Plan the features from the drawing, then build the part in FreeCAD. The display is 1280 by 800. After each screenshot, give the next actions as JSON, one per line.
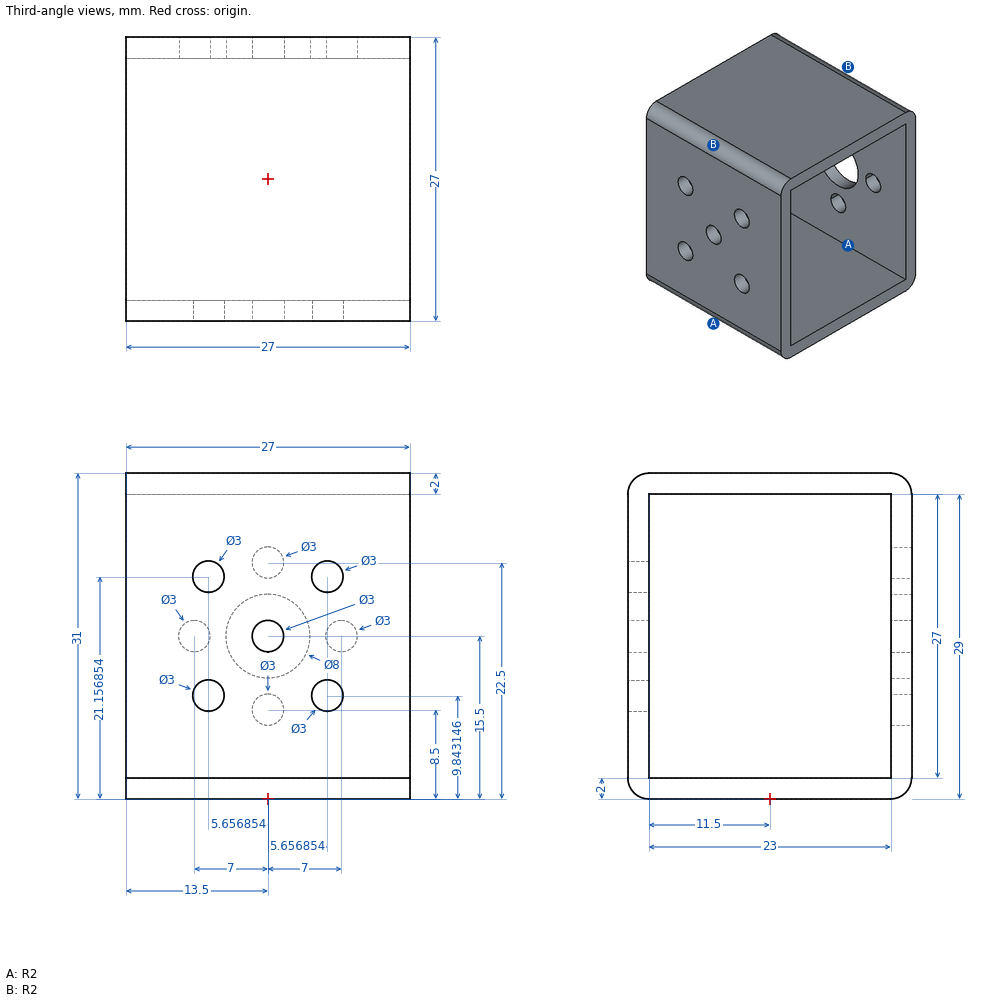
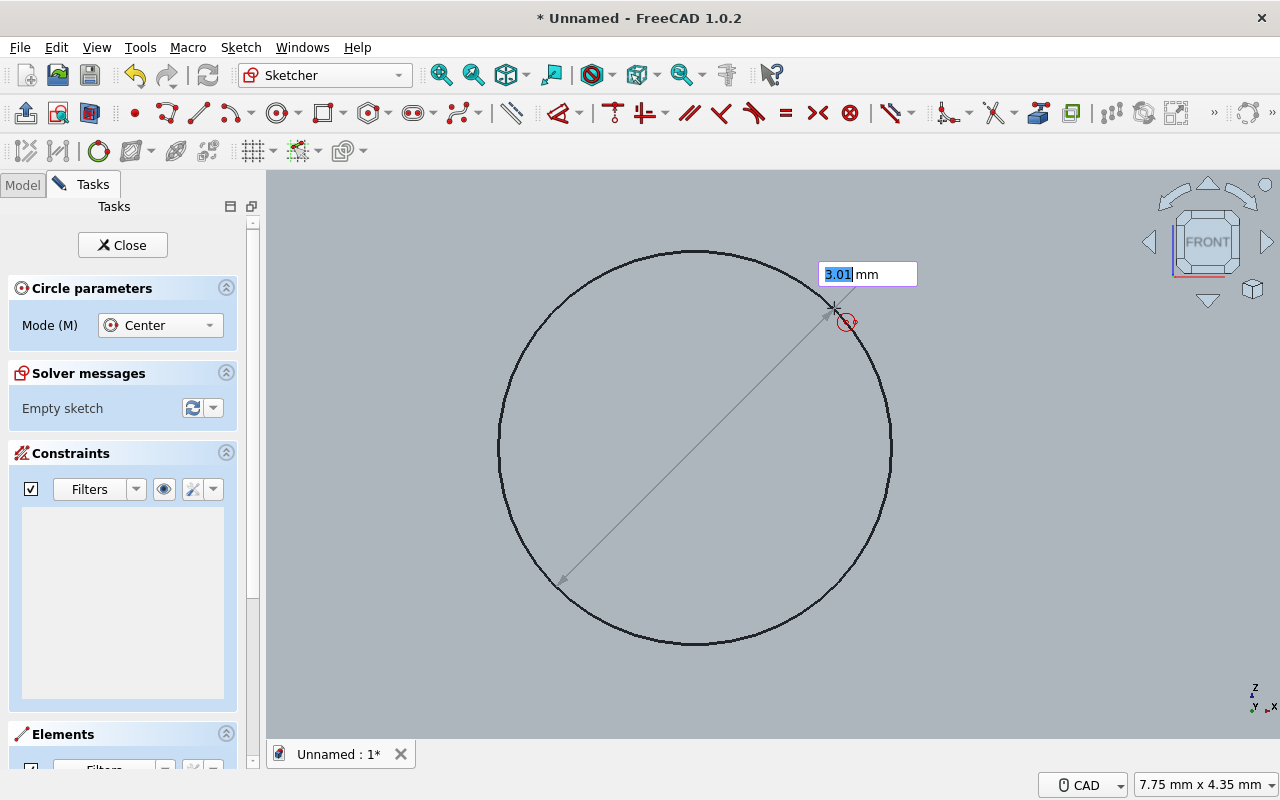
{"action": "type", "text": "3"}
{"action": "key", "text": "Return"}
{"action": "key", "text": "Escape"}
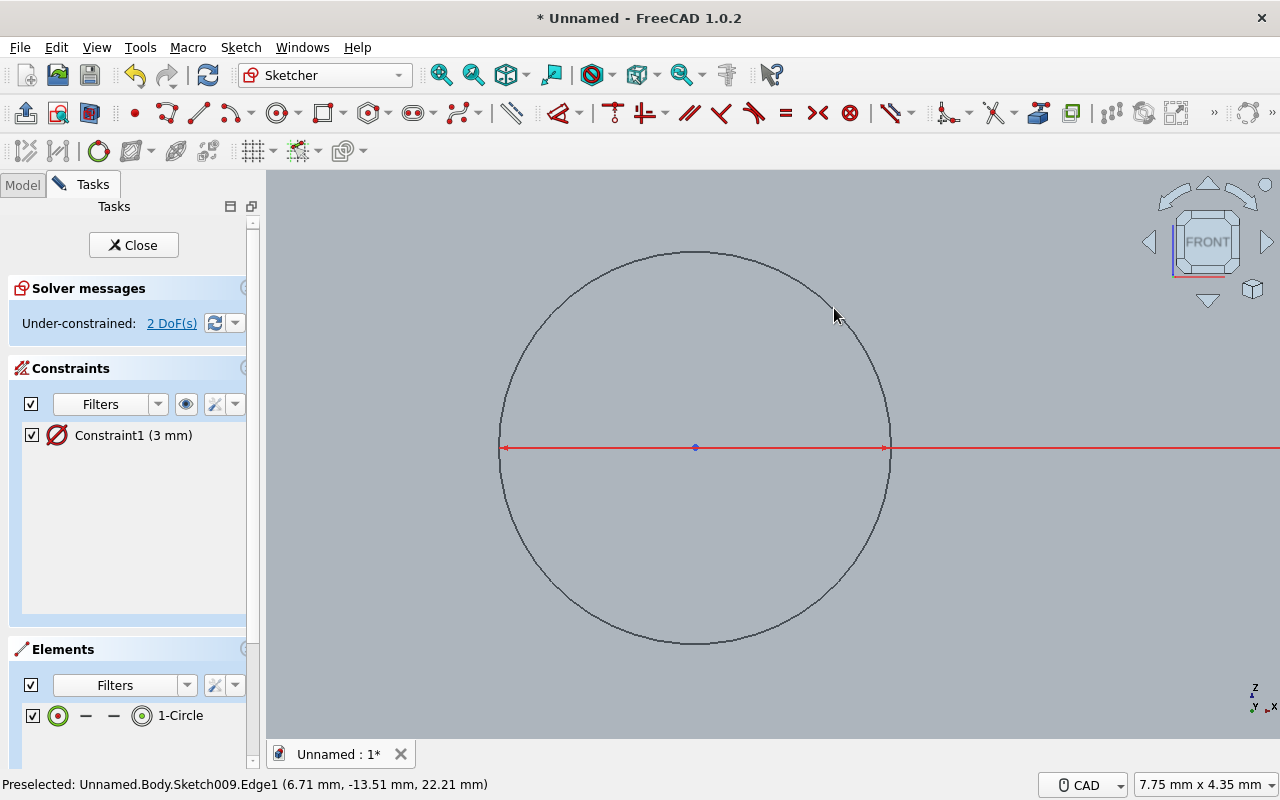
{"action": "left_click", "coordinate": [558, 114]}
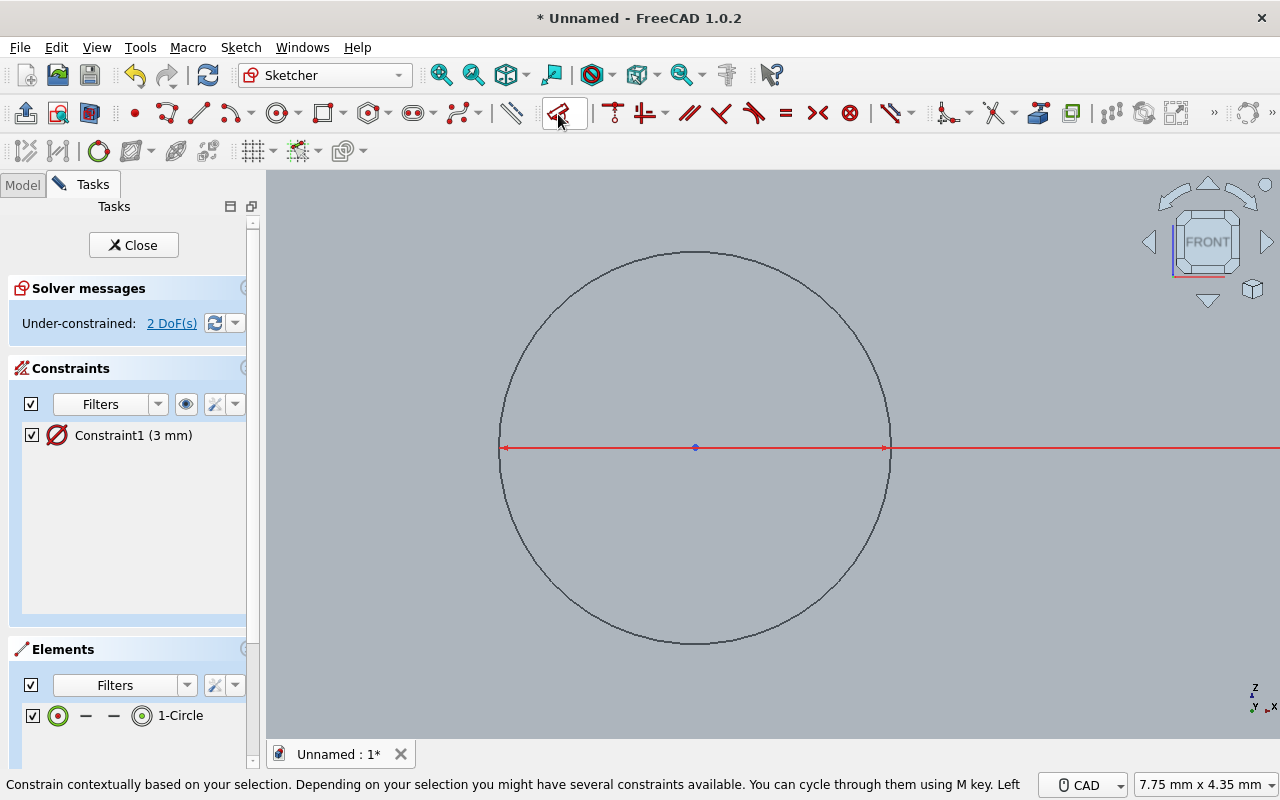
{"action": "left_click", "coordinate": [695, 448]}
{"action": "left_click", "coordinate": [402, 414]}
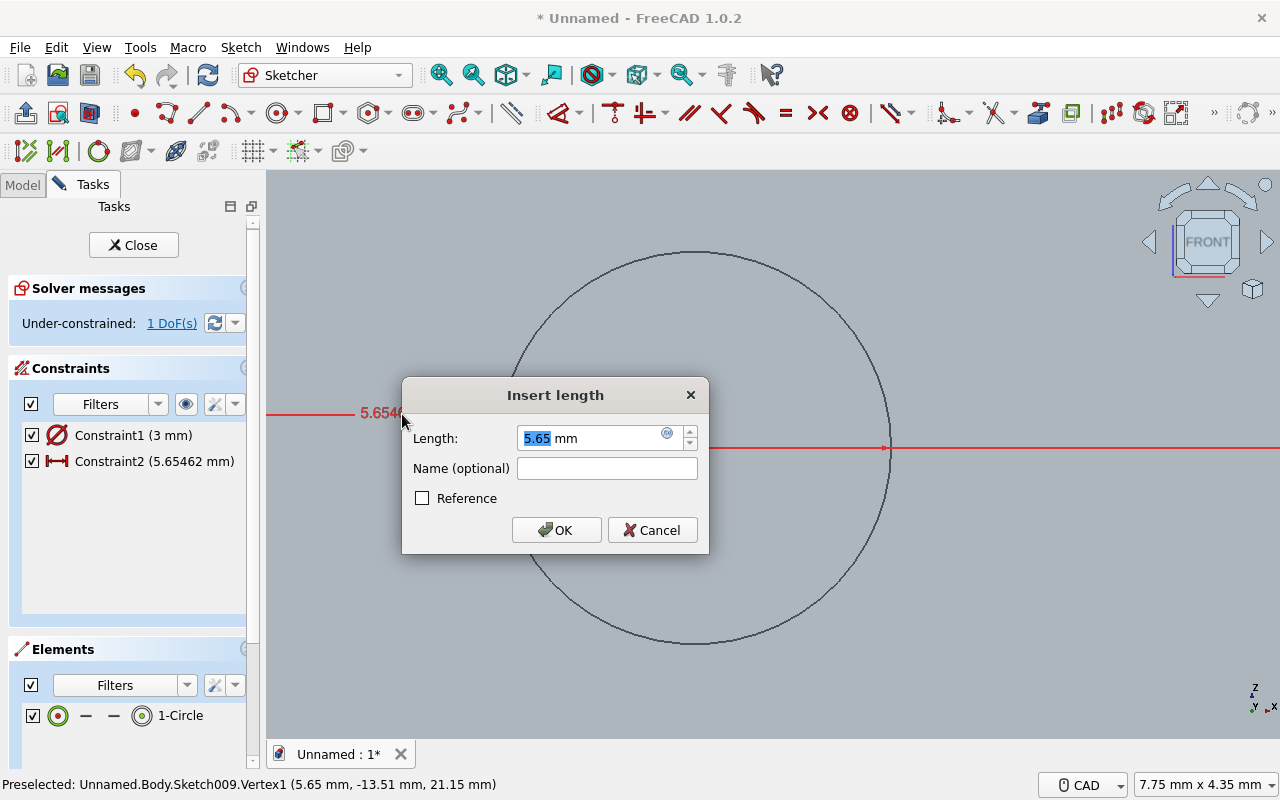
{"action": "type", "text": "5.656854"}
{"action": "key", "text": "Return"}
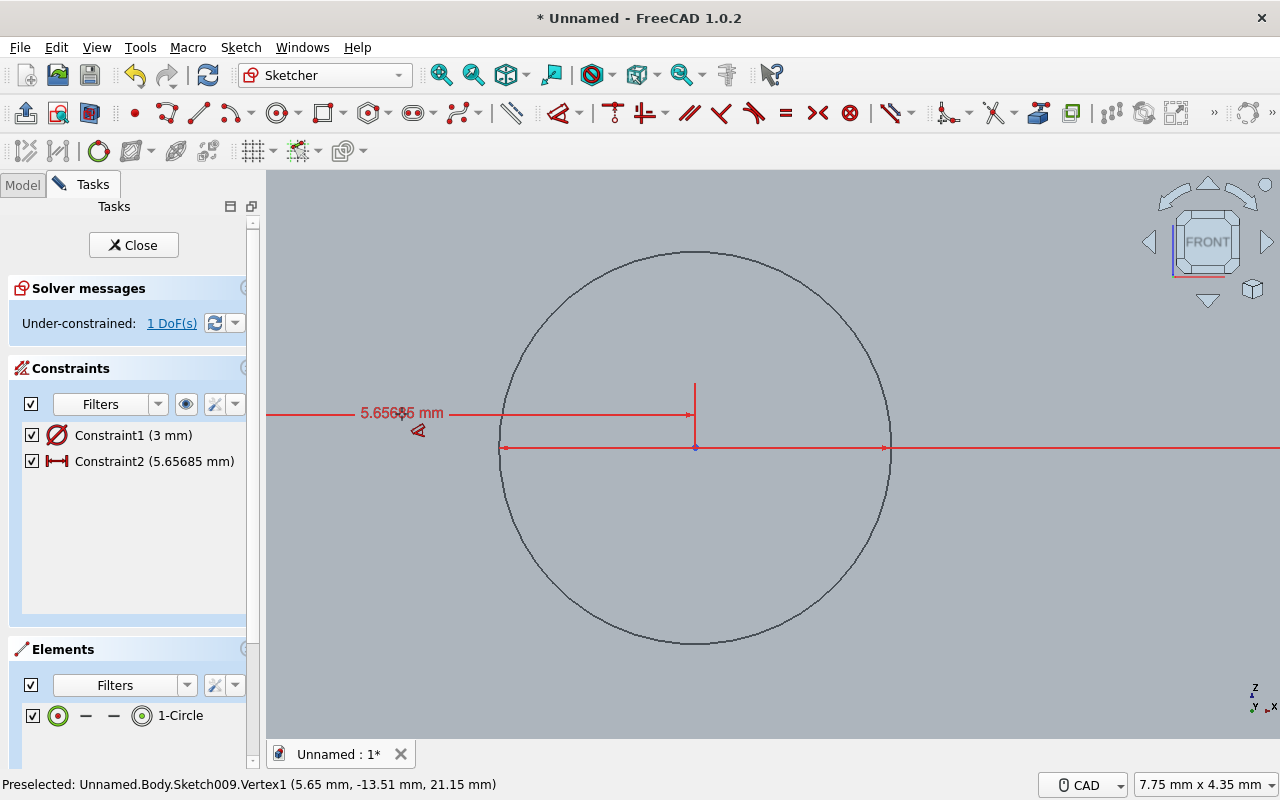
{"action": "left_click", "coordinate": [695, 448]}
{"action": "left_click", "coordinate": [729, 579]}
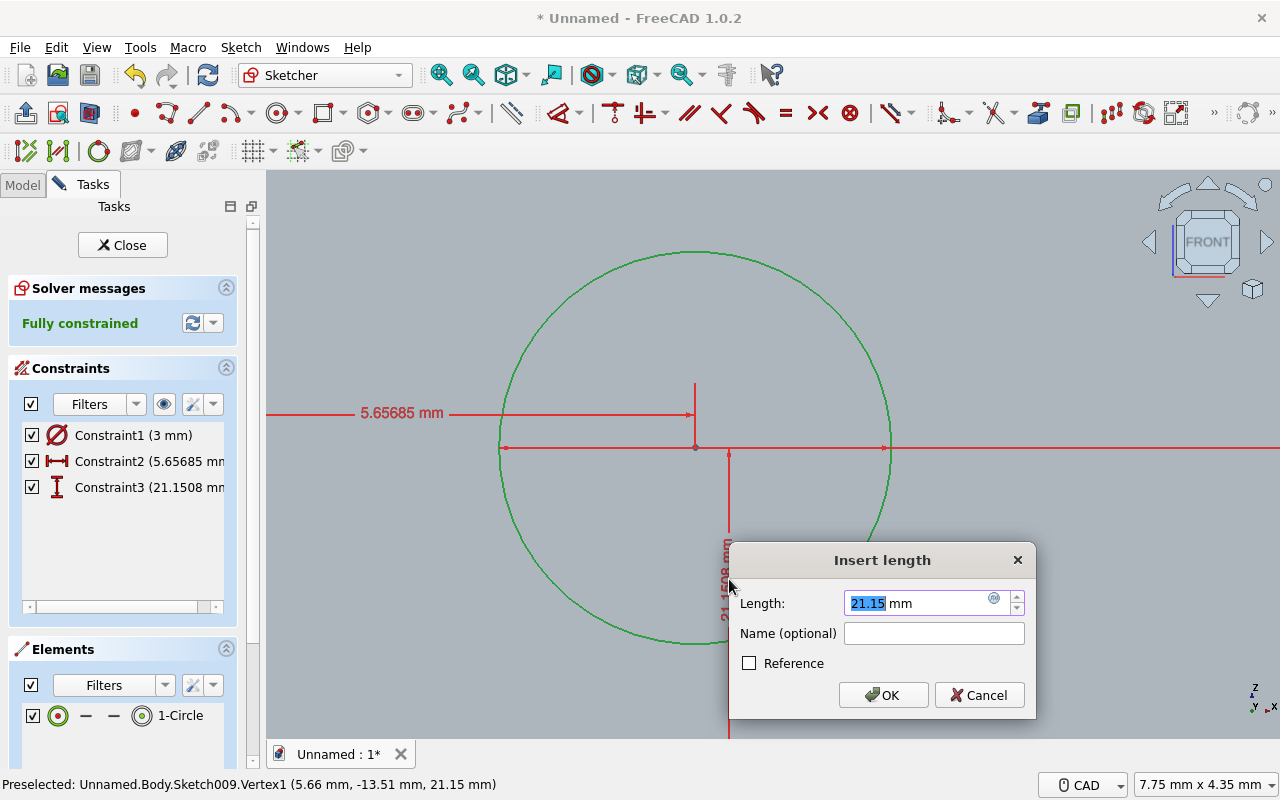
{"action": "type", "text": "21.156854"}
{"action": "key", "text": "Return"}
{"action": "key", "text": "Escape"}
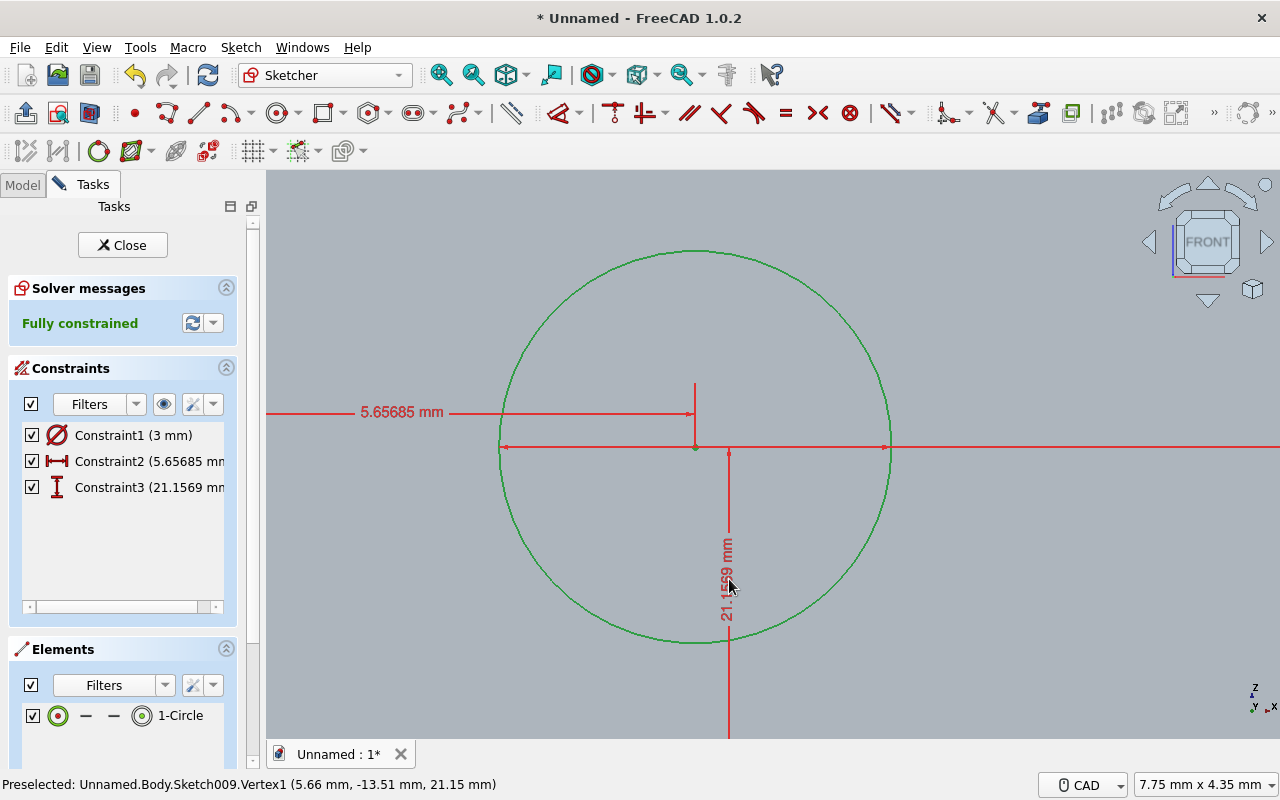
{"action": "left_click", "coordinate": [123, 245]}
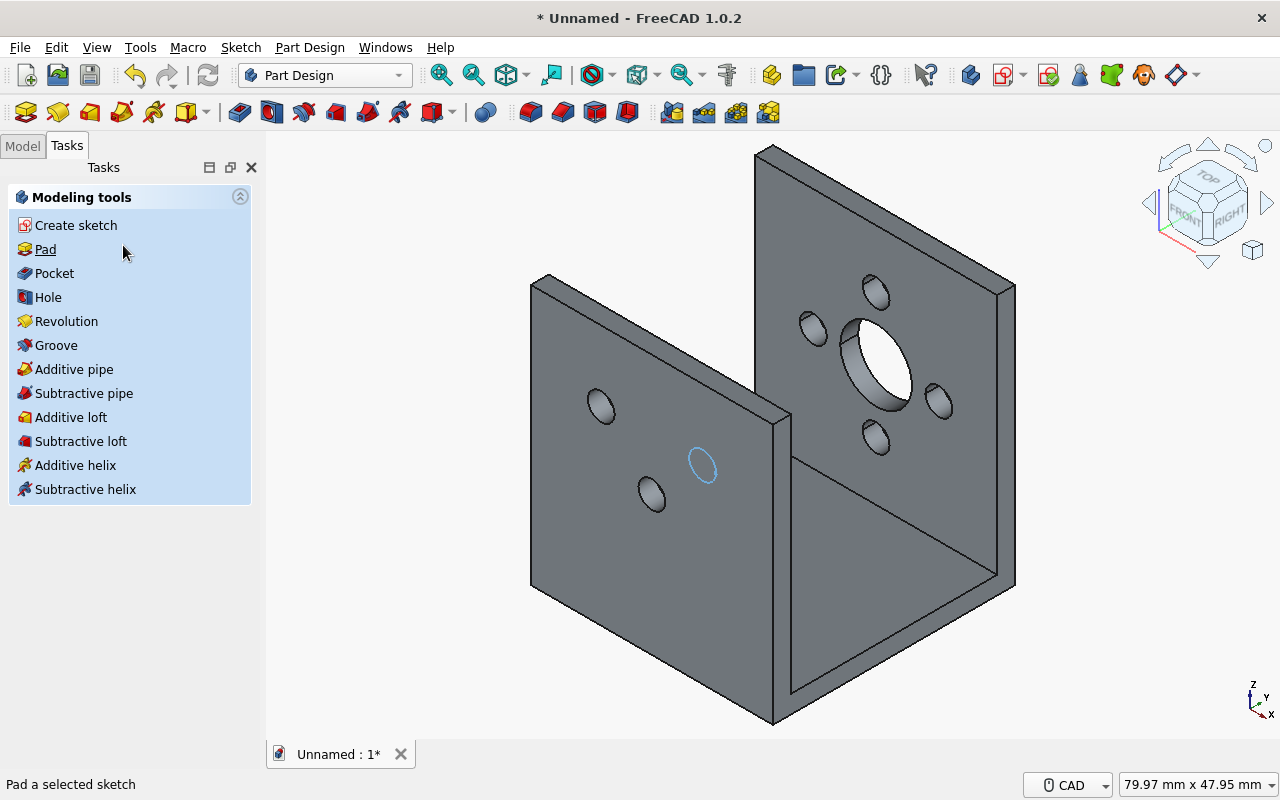
{"action": "left_click", "coordinate": [240, 112]}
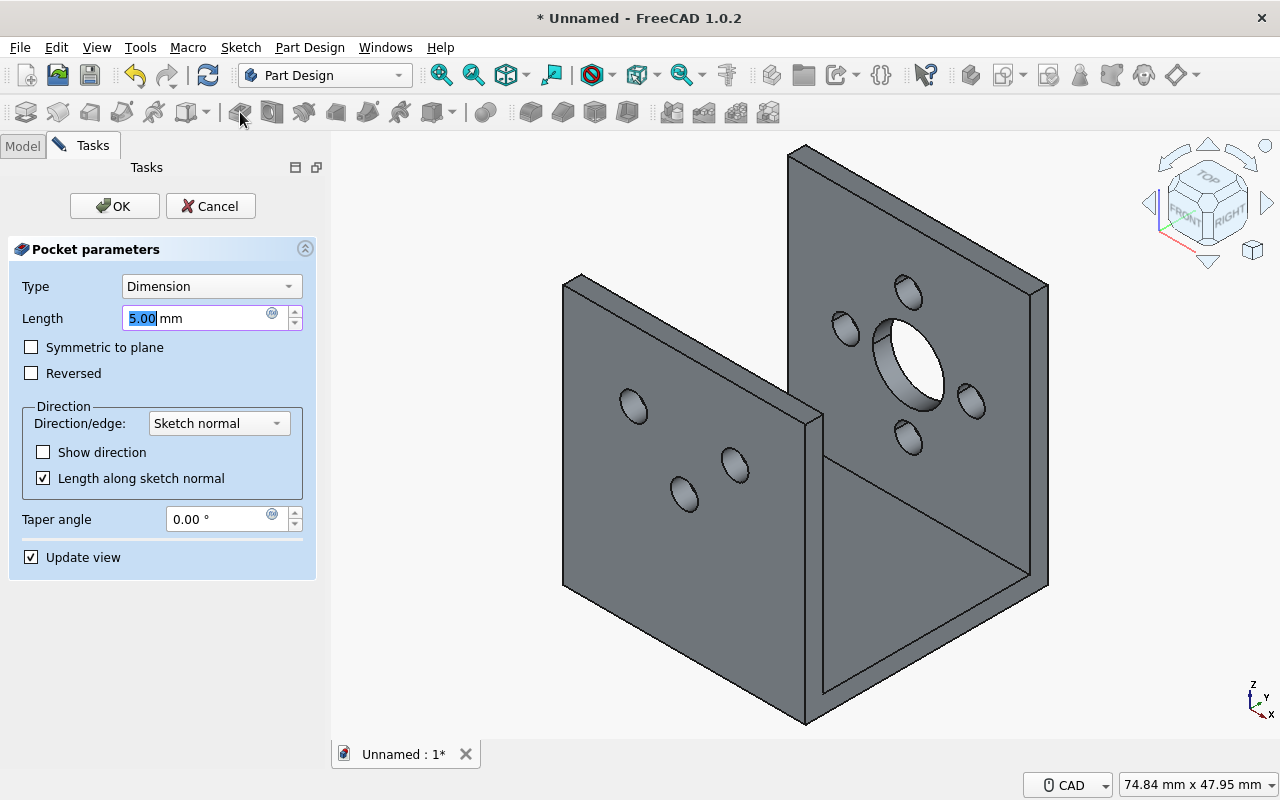
{"action": "left_click", "coordinate": [212, 286]}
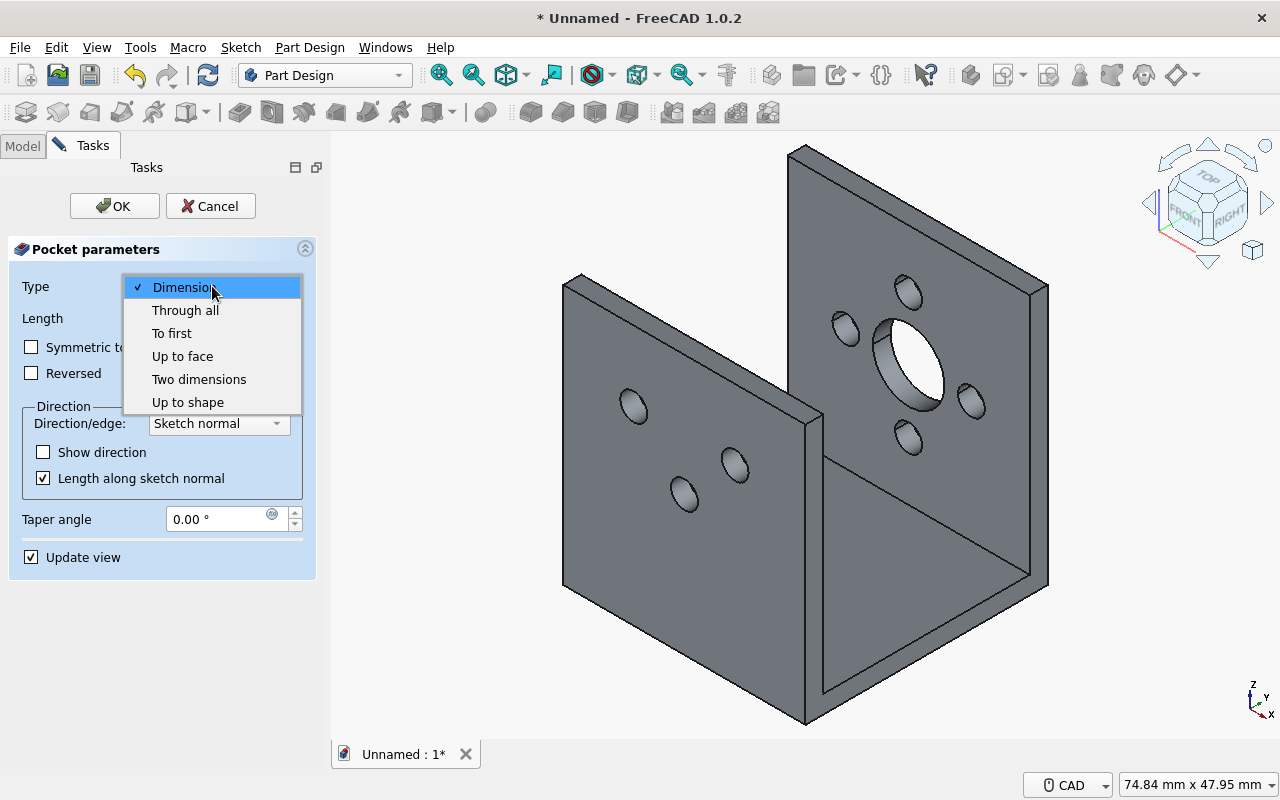
{"action": "left_click", "coordinate": [212, 334]}